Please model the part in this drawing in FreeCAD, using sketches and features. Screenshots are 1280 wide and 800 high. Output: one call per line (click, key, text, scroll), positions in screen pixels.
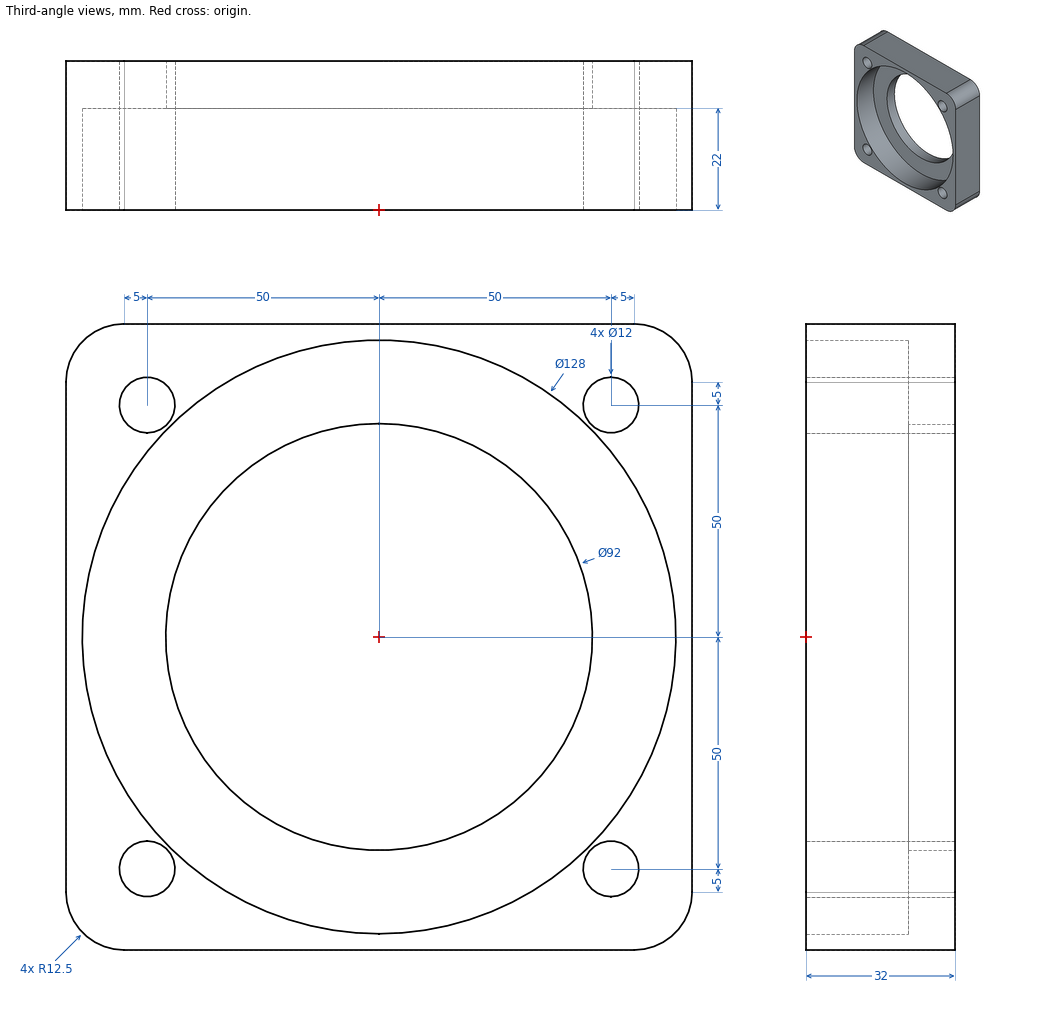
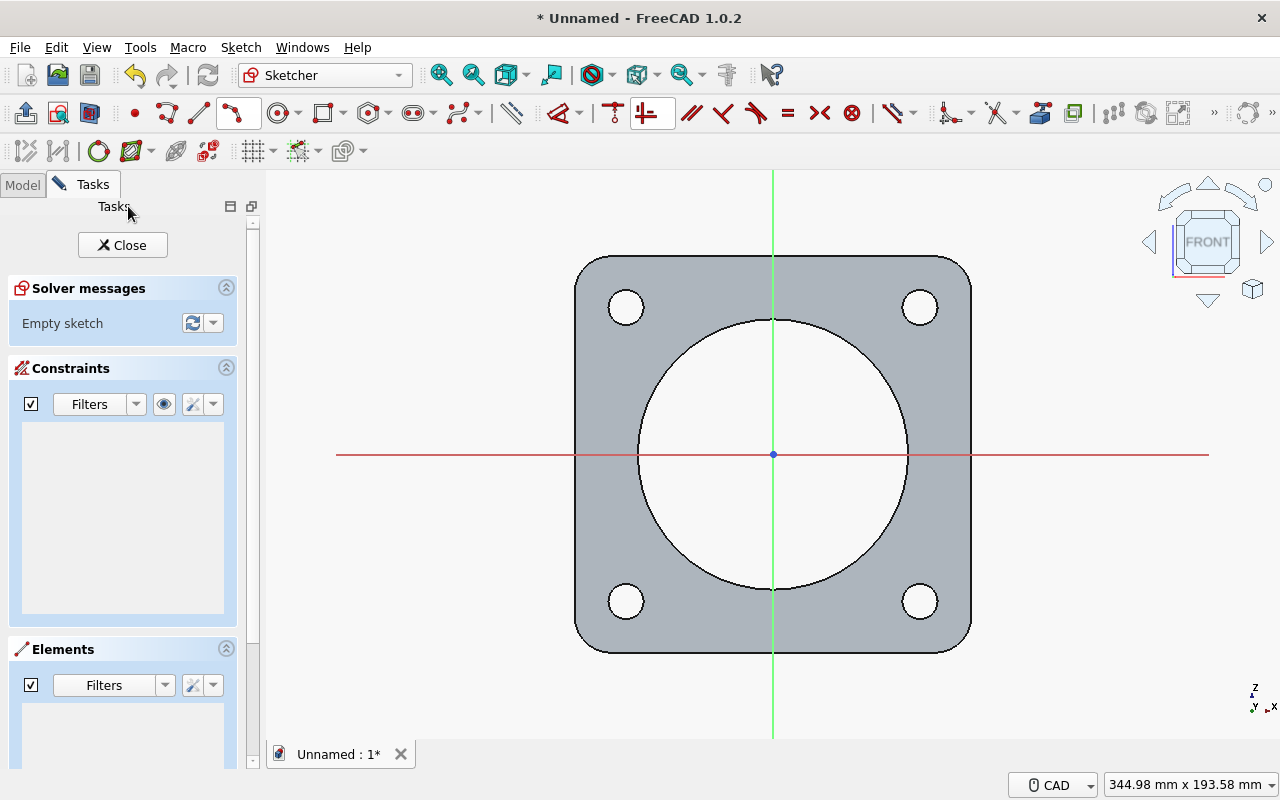
click(278, 114)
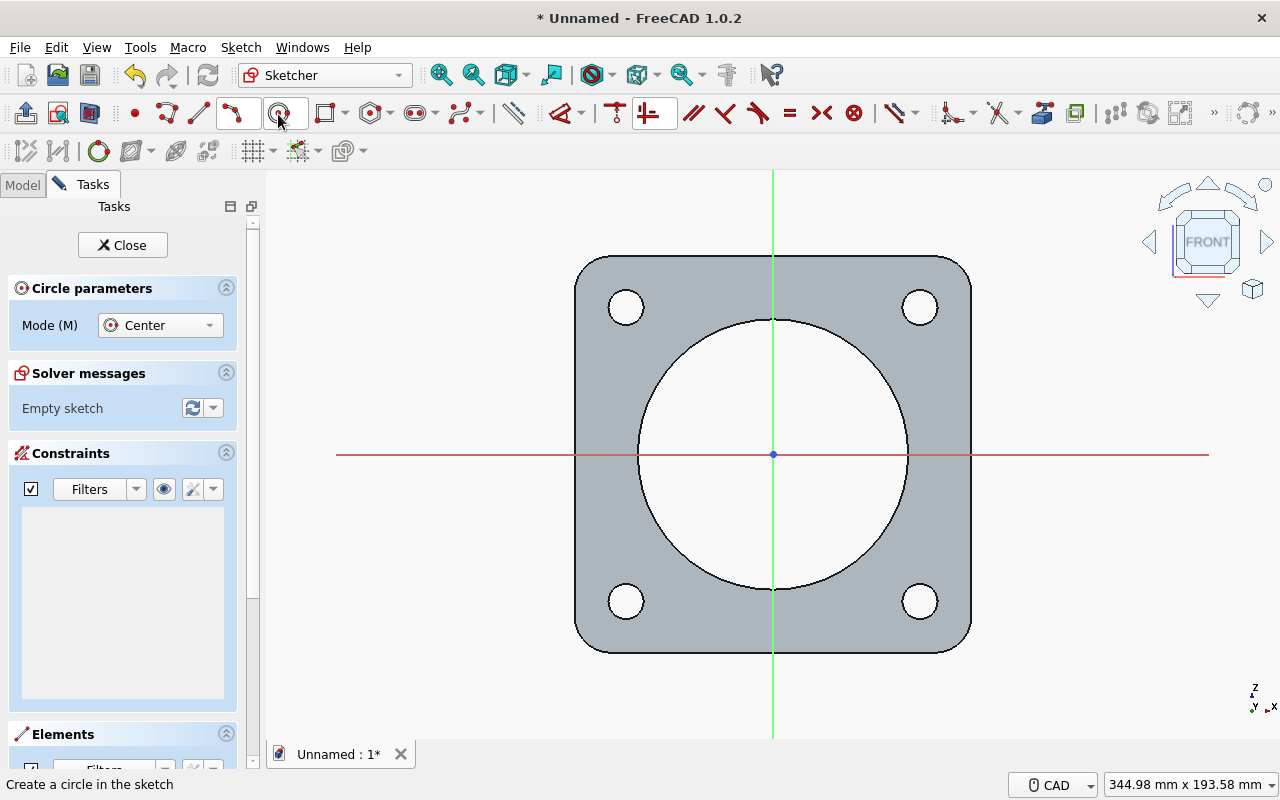
click(773, 455)
click(906, 321)
key(Escape)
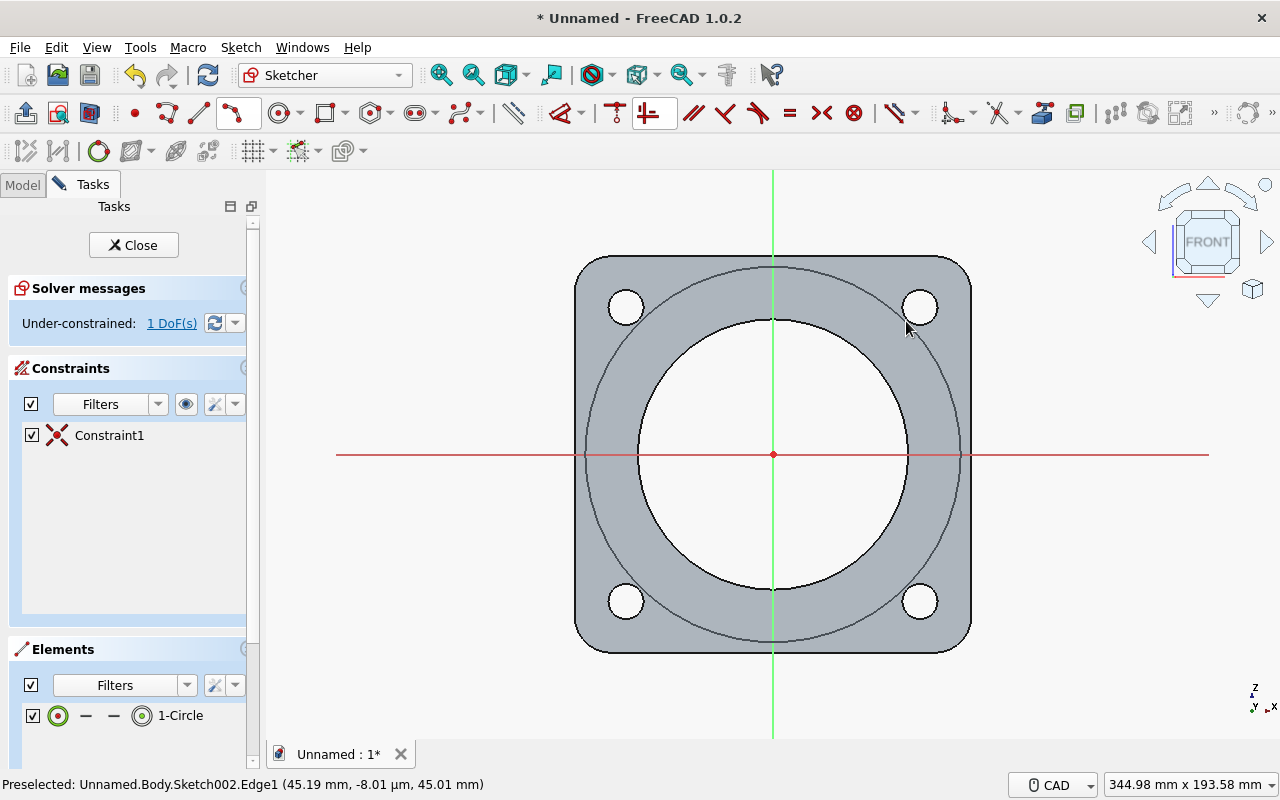
click(560, 114)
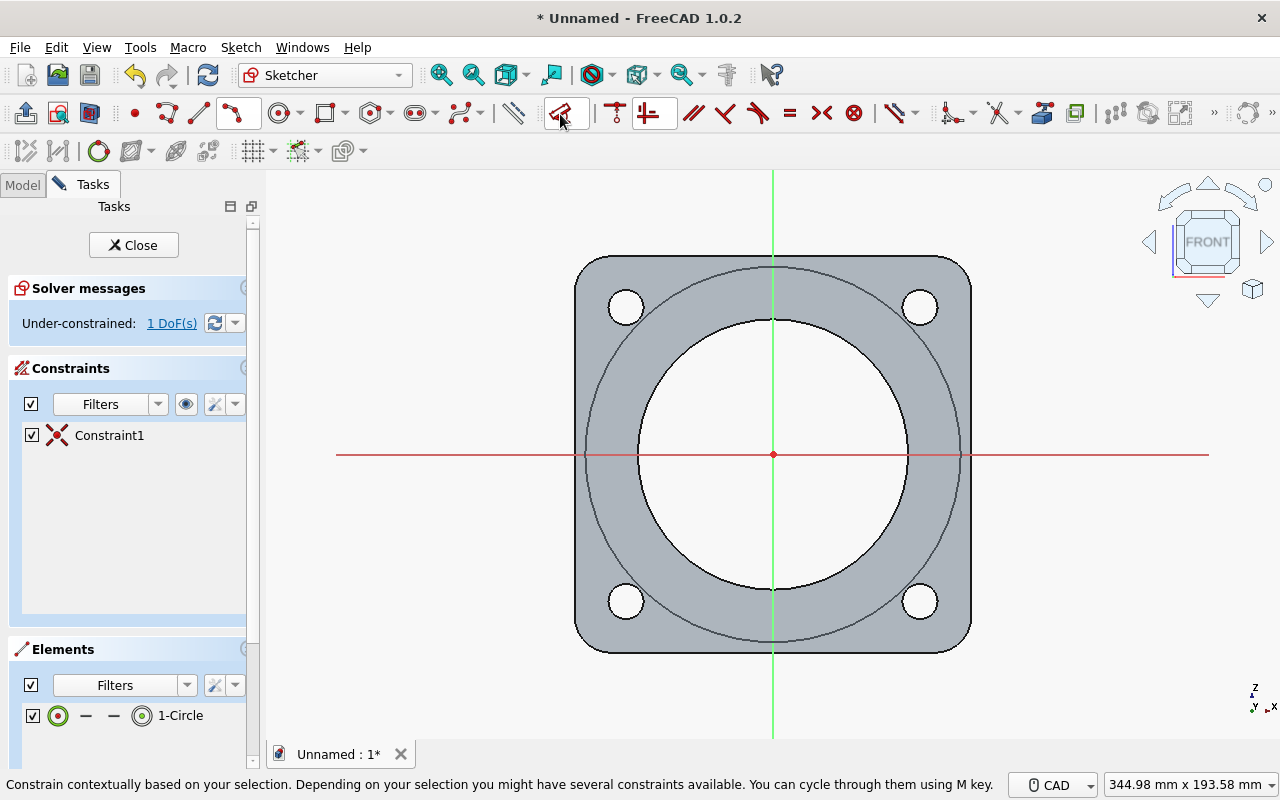
click(905, 321)
click(927, 298)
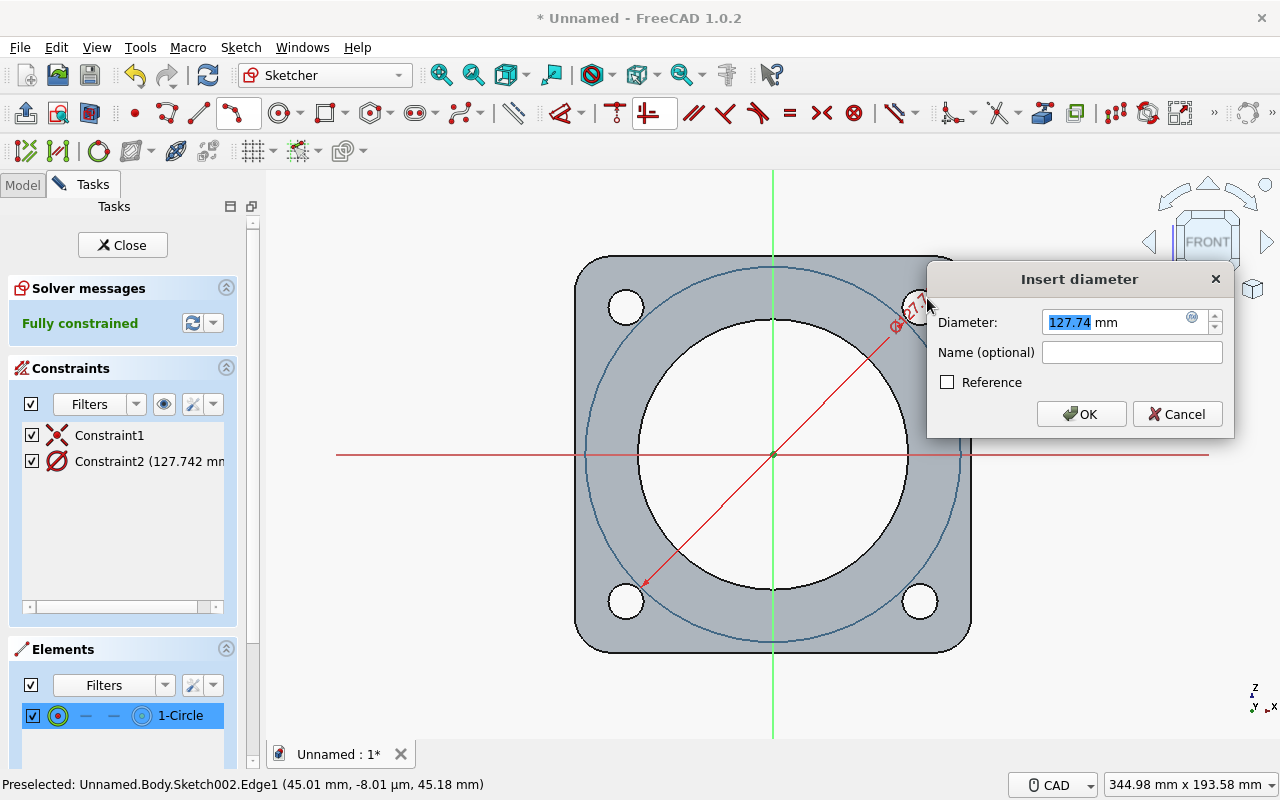
text(128)
key(Return)
key(Escape)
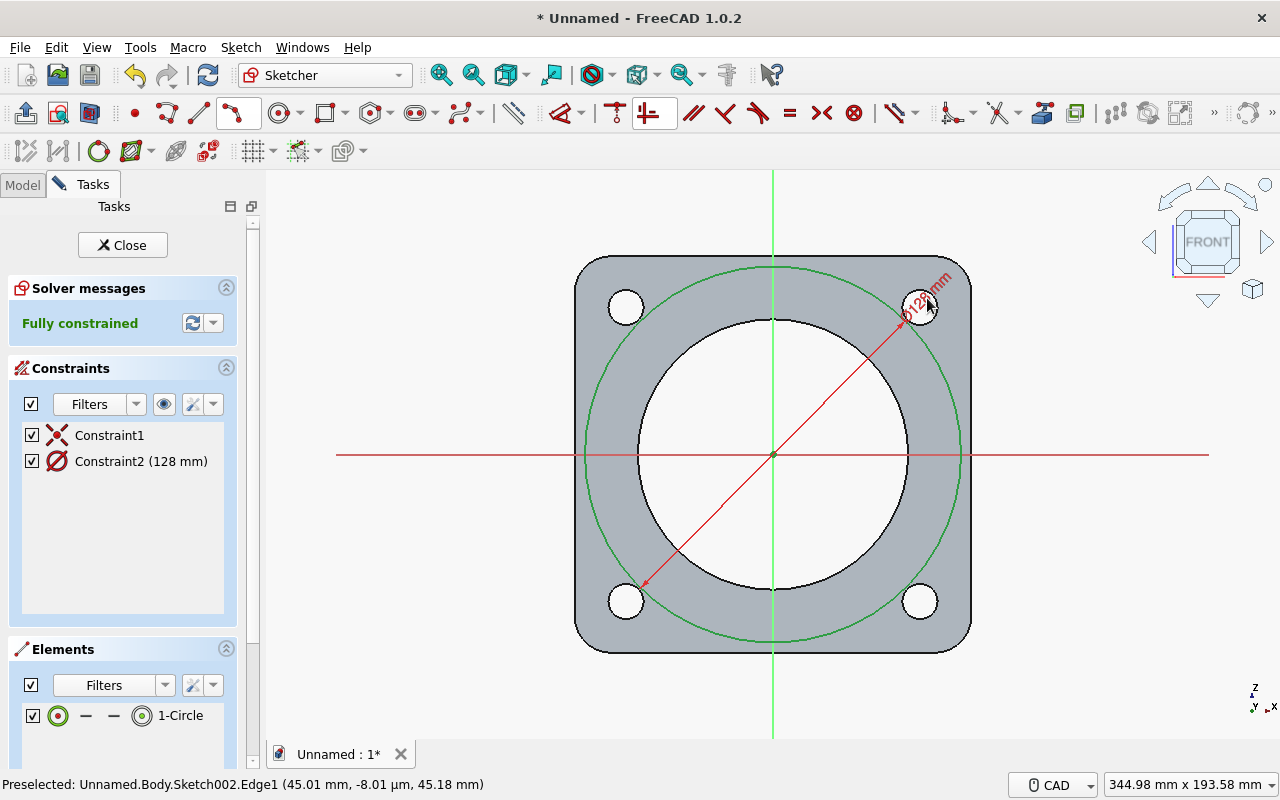
click(123, 245)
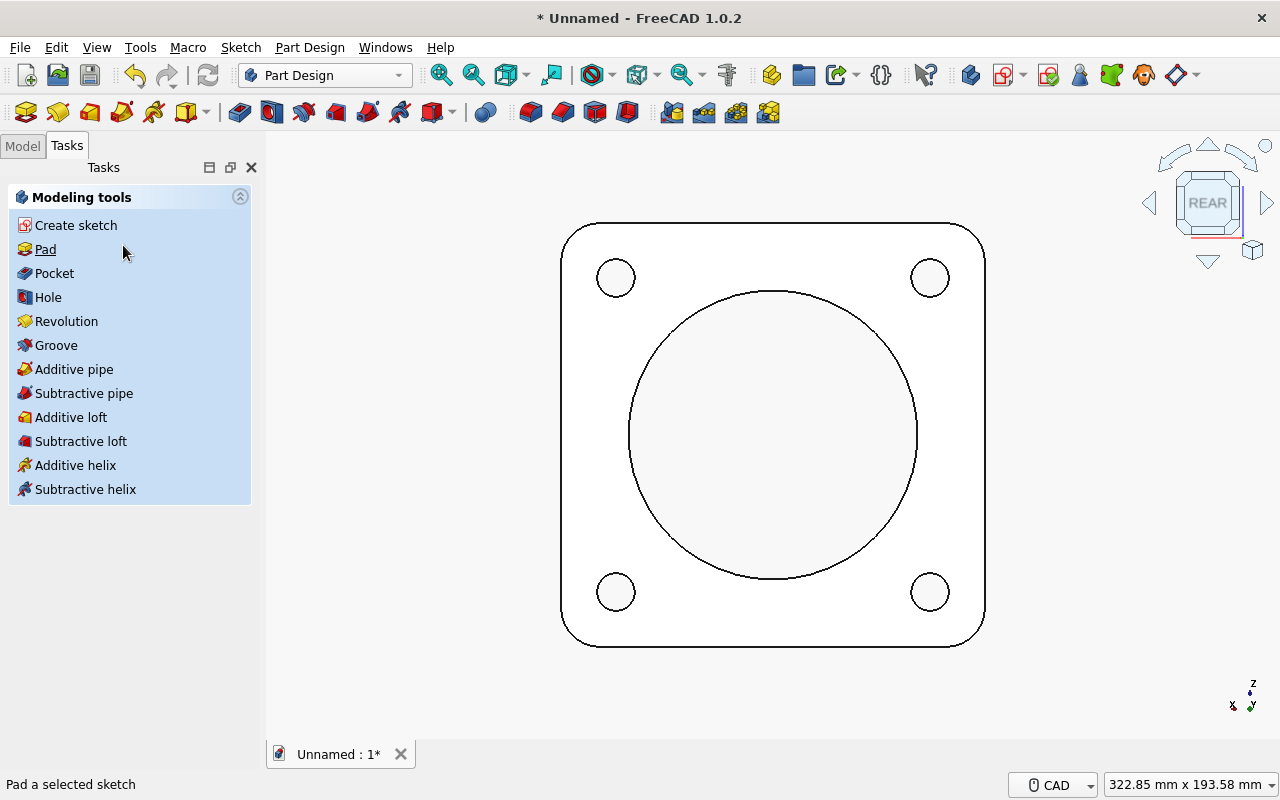
click(240, 112)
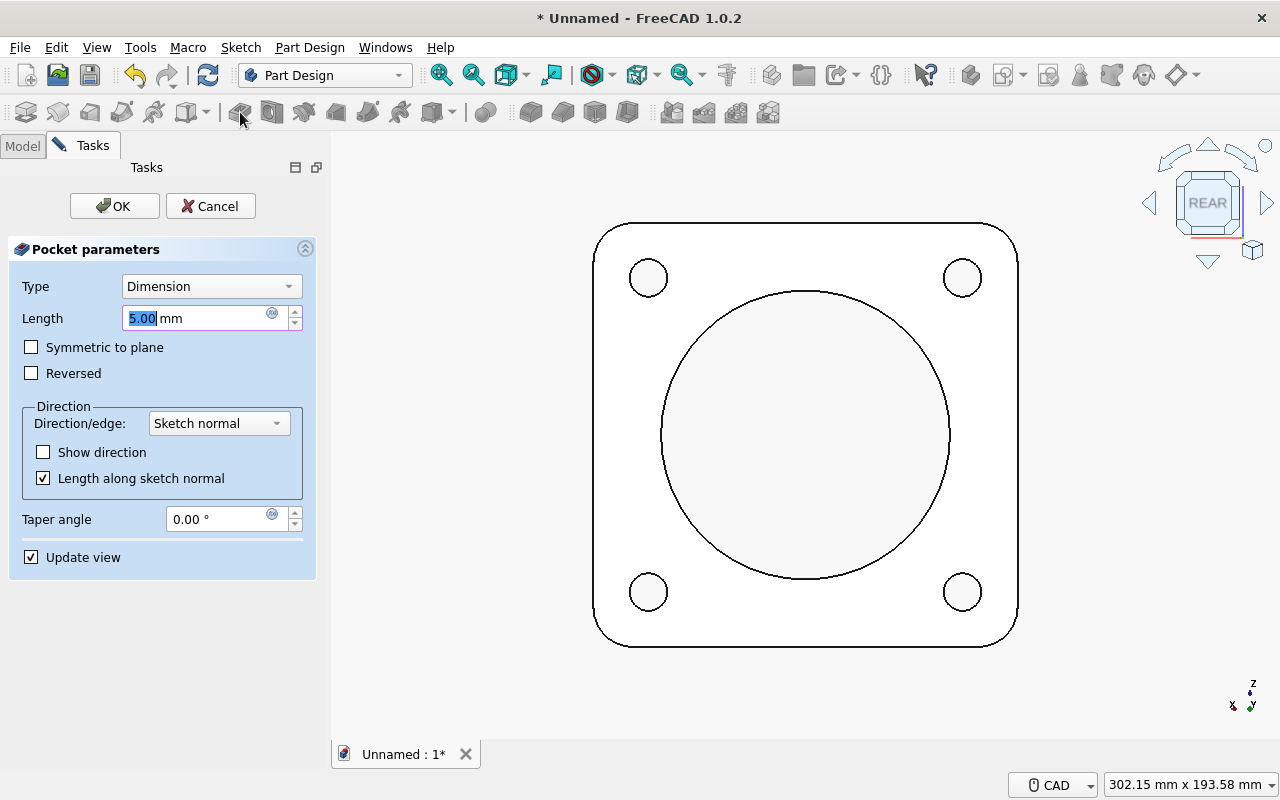
text(22)
key(Tab)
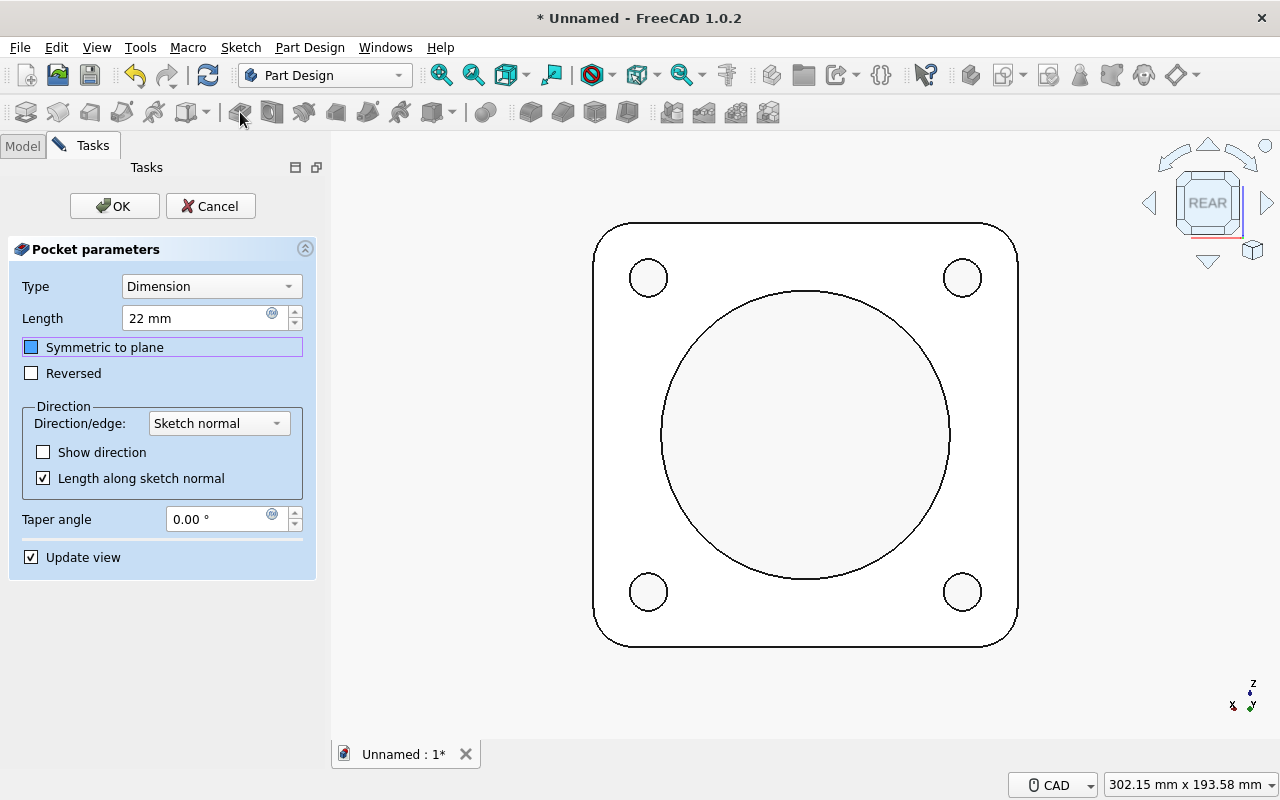
click(115, 206)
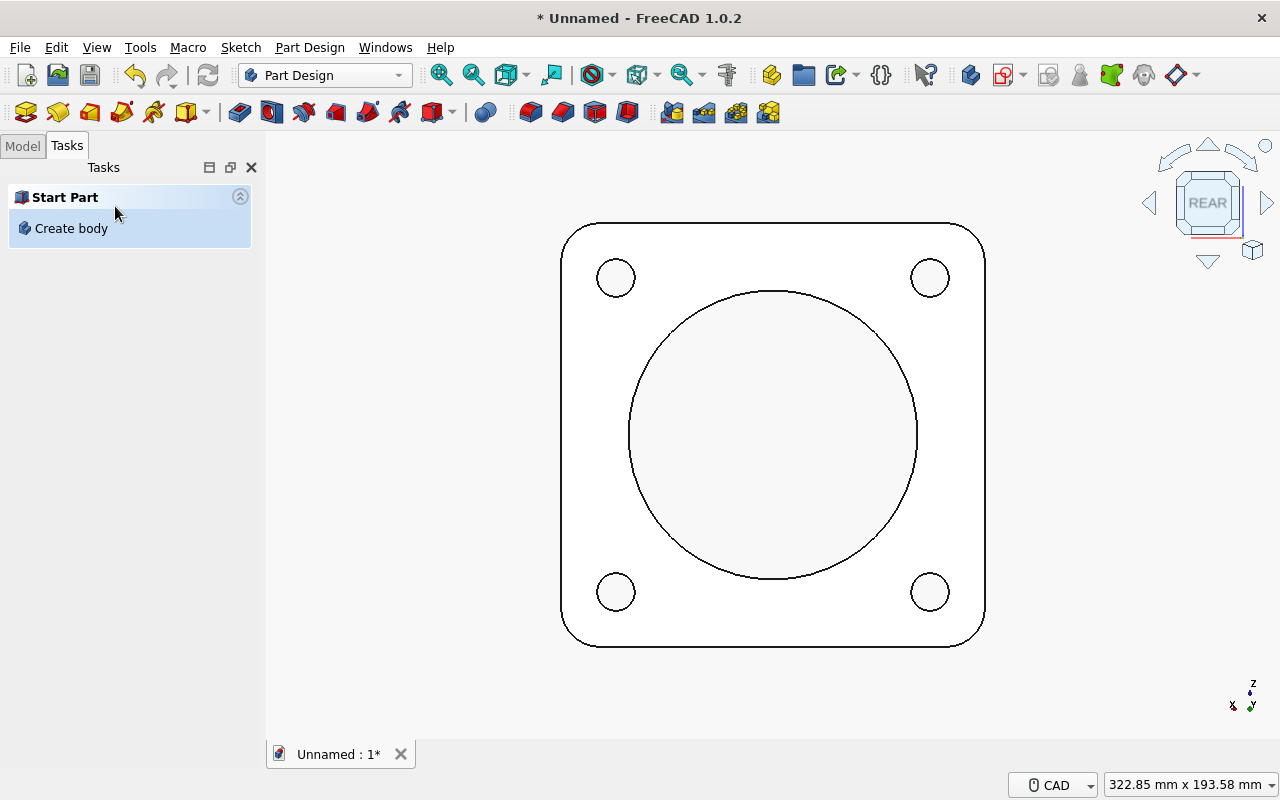
key(0)